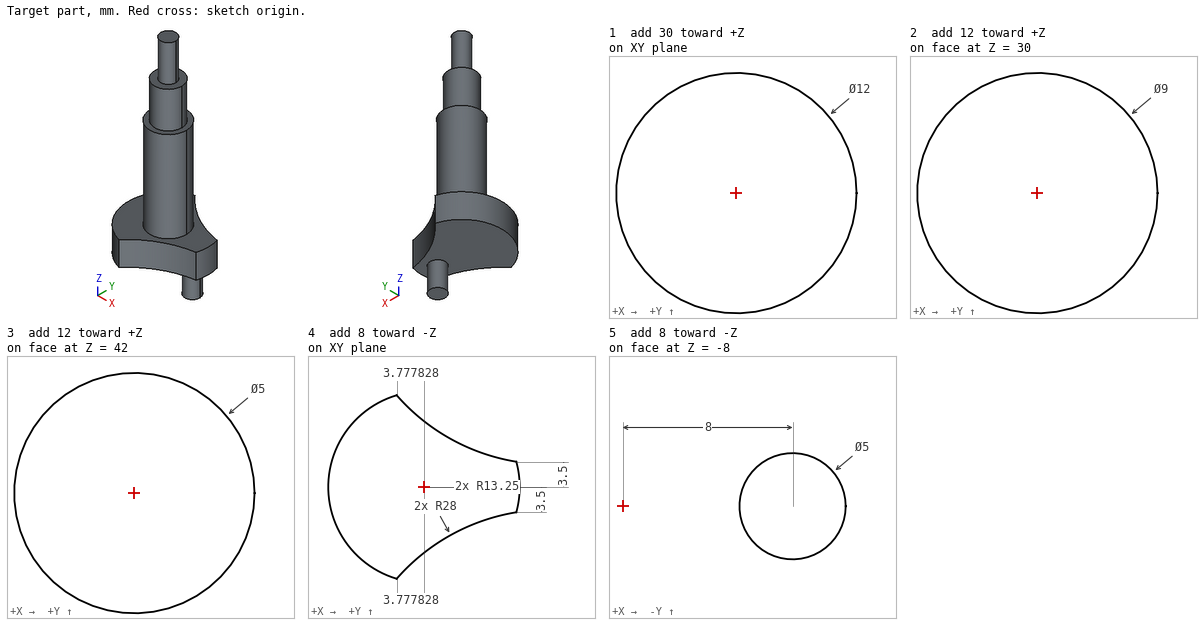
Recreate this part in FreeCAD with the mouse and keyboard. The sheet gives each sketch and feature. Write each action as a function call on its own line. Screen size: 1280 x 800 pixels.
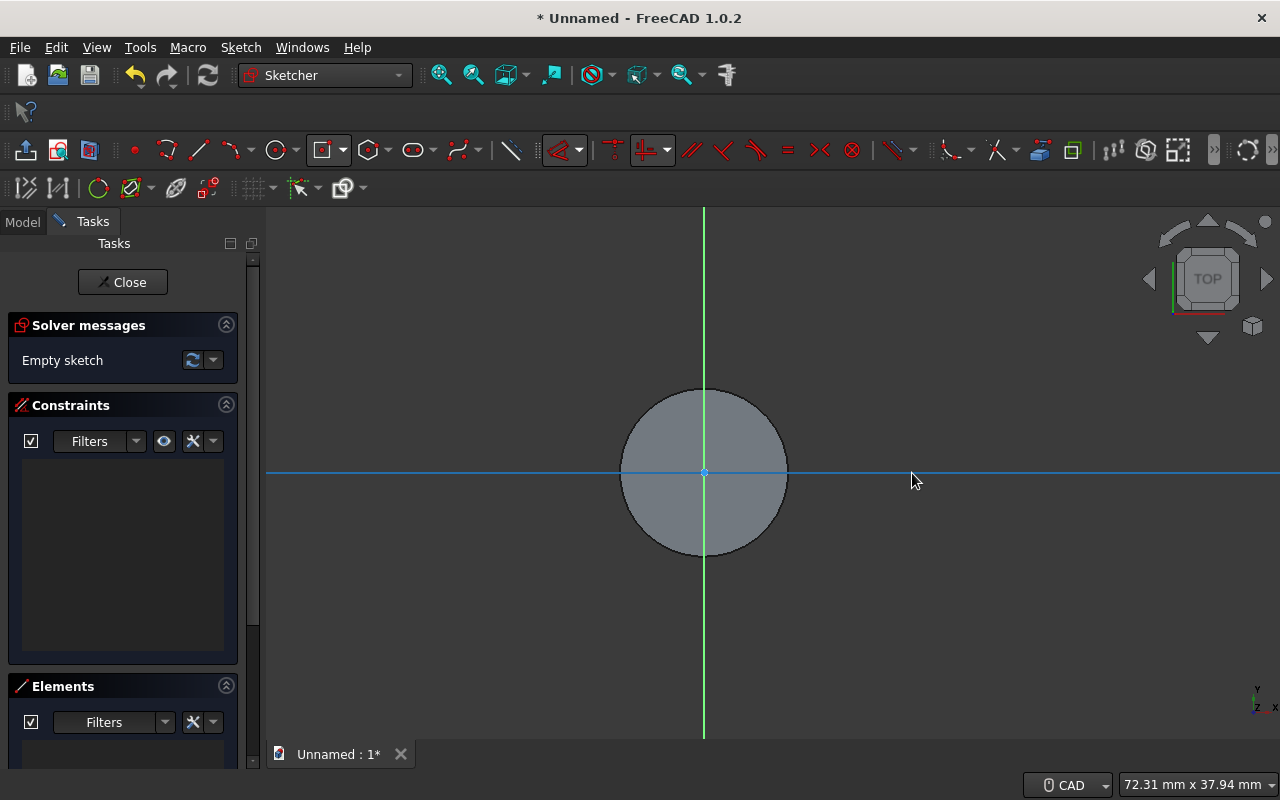
click(232, 150)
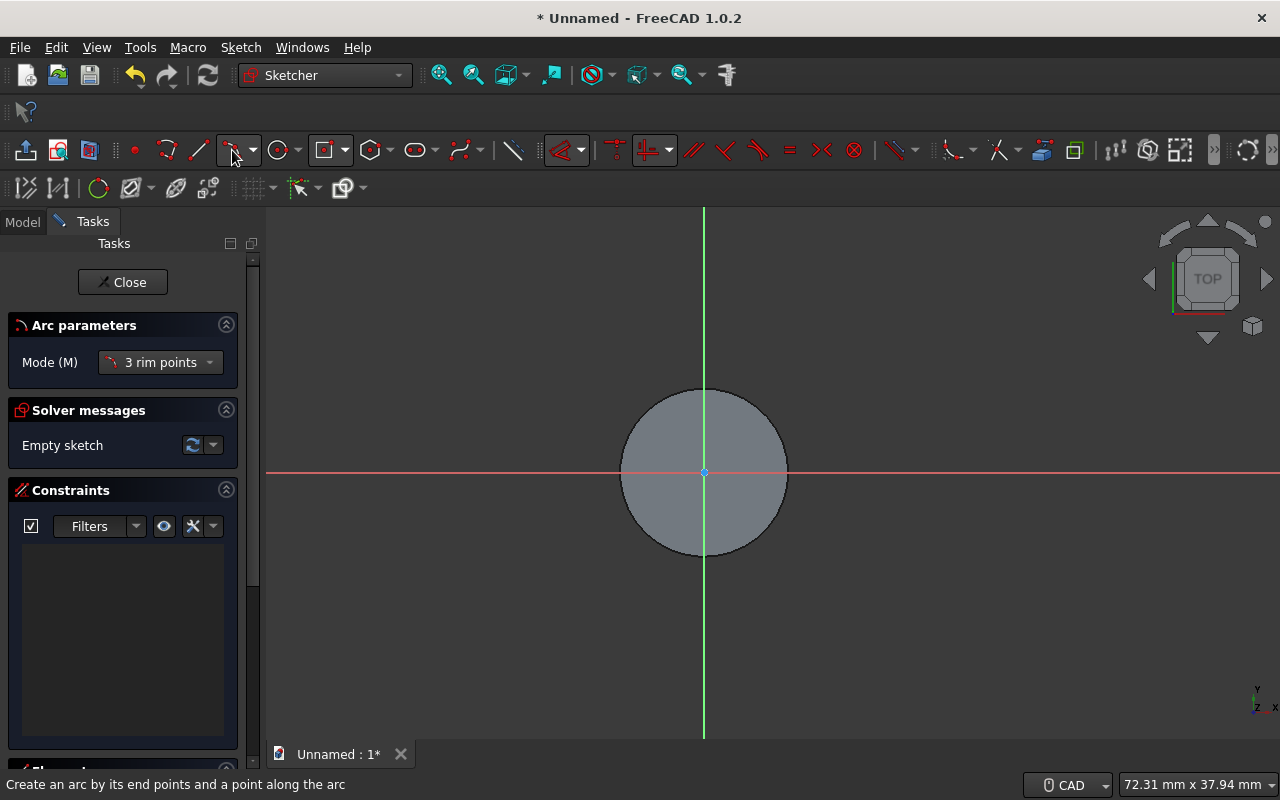
click(651, 651)
click(651, 295)
click(524, 426)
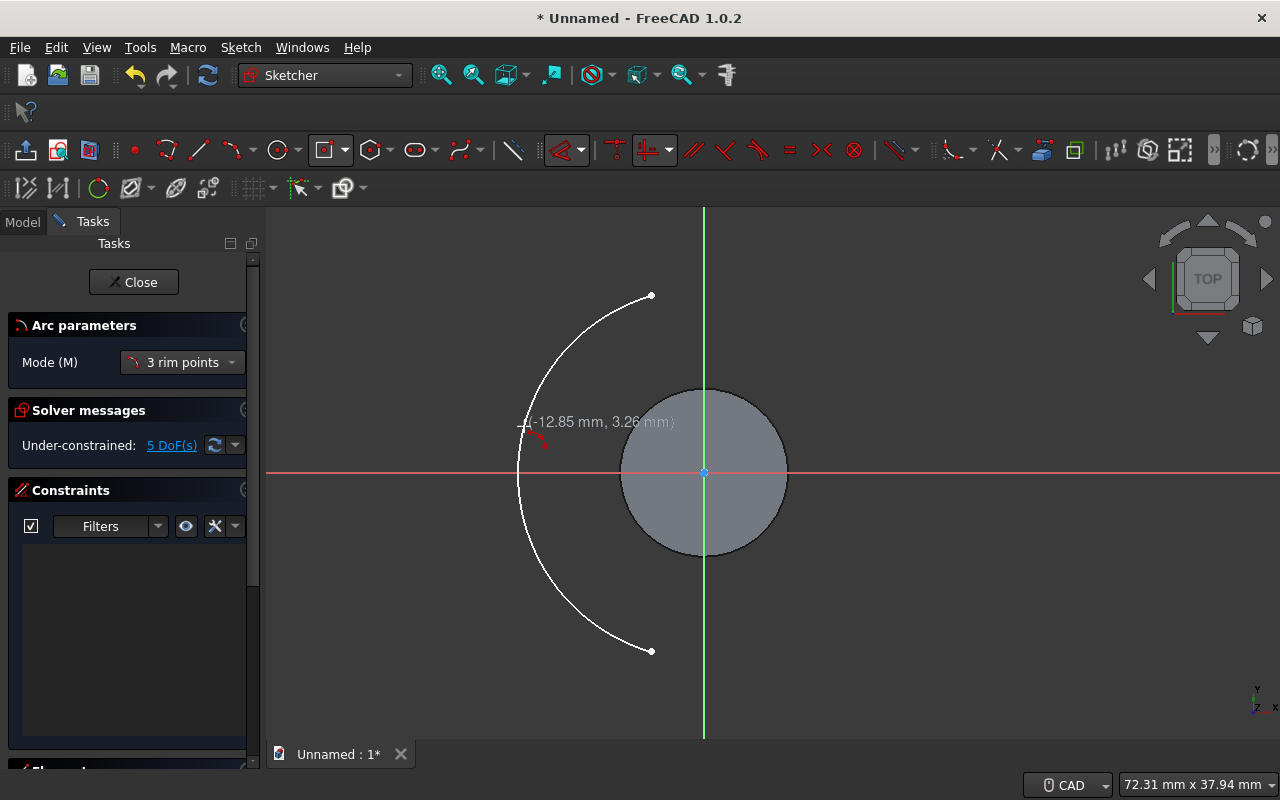
click(651, 296)
click(883, 424)
click(756, 379)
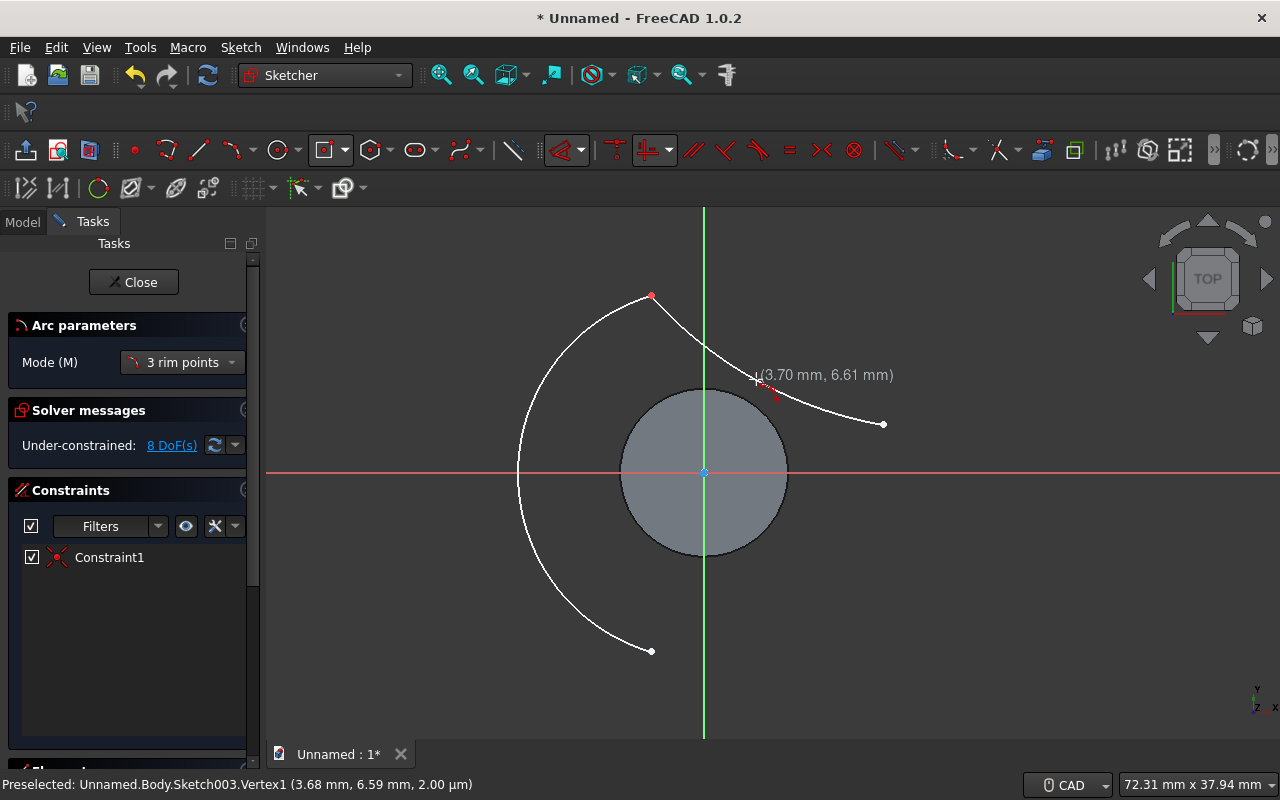
click(883, 425)
click(883, 522)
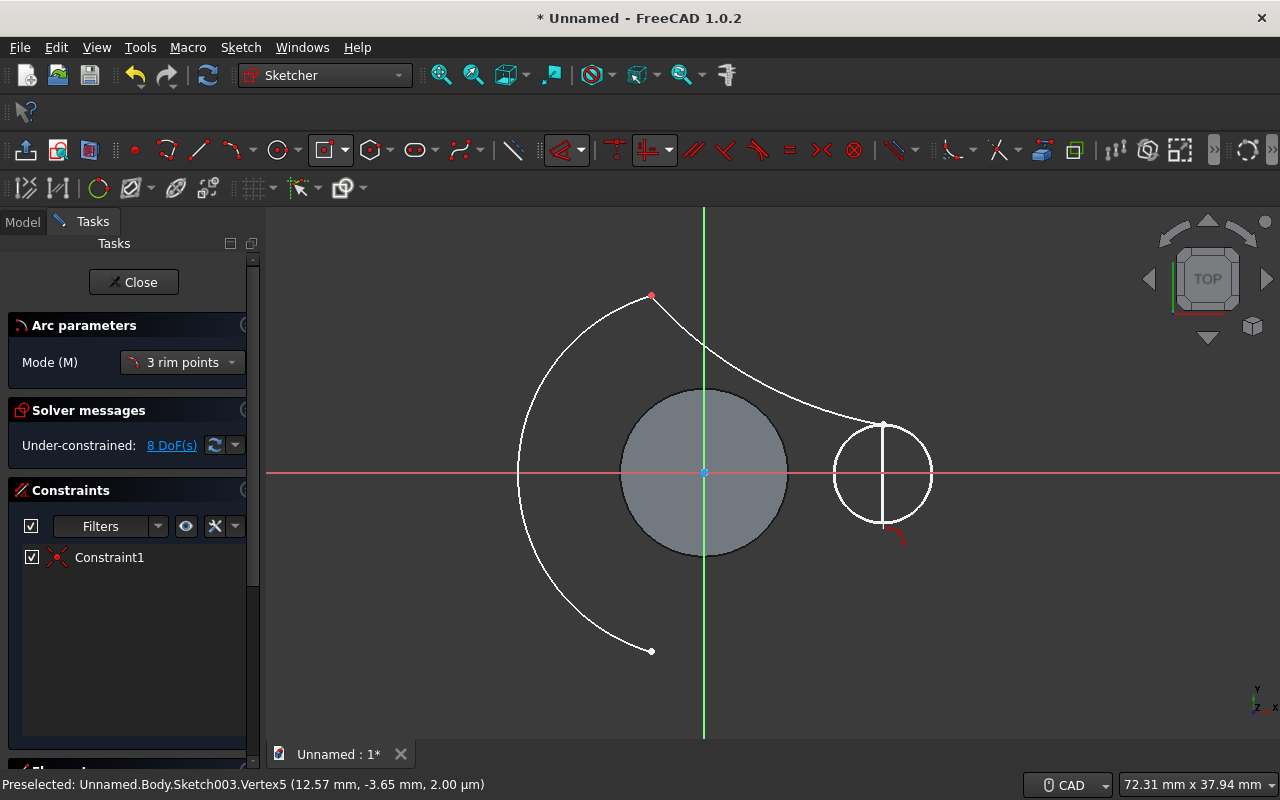
scroll(890, 483, up, 5)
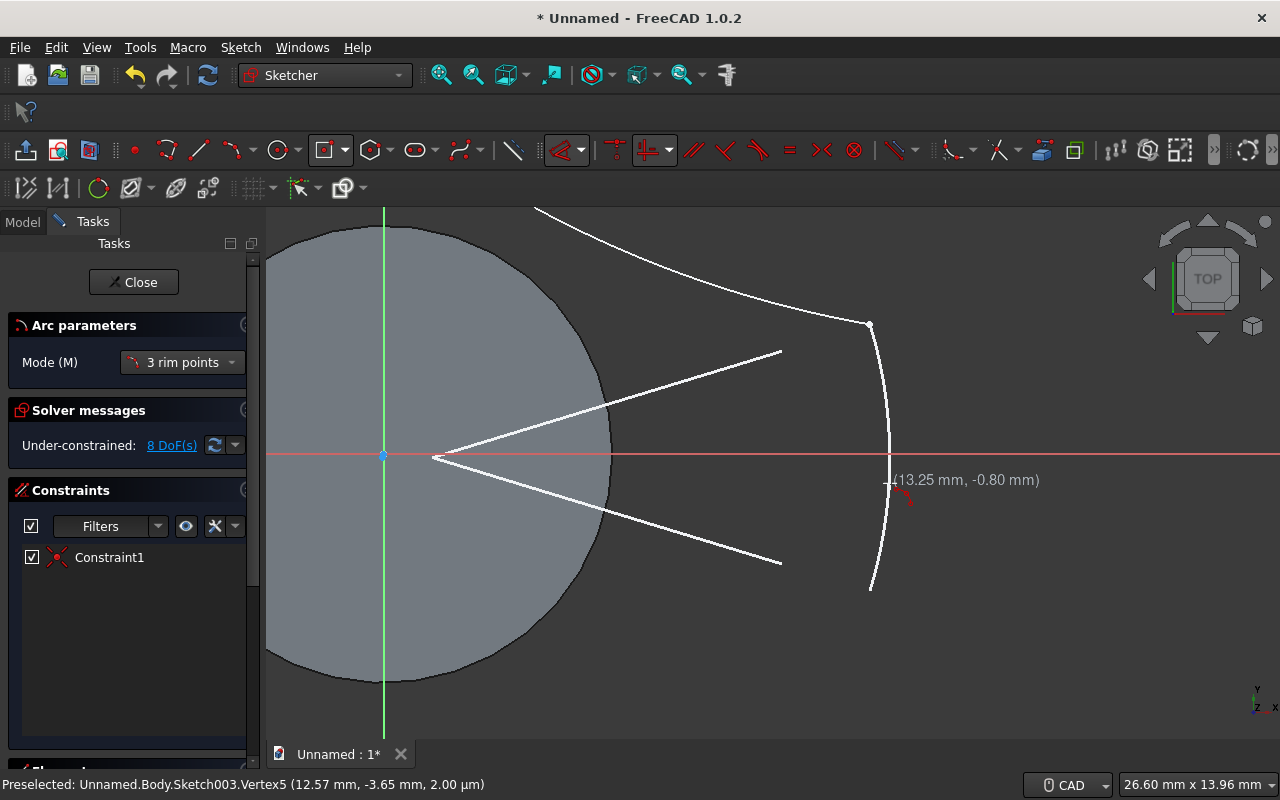
click(888, 481)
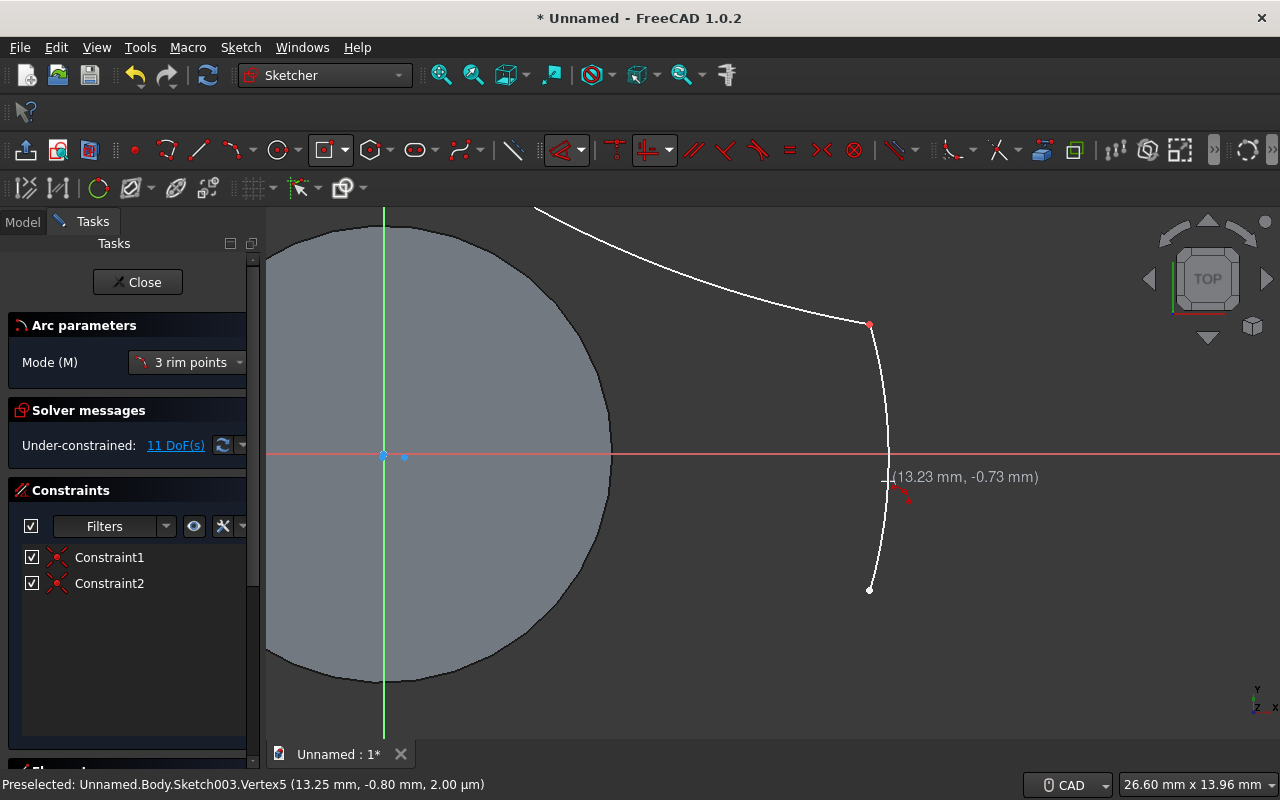
click(870, 591)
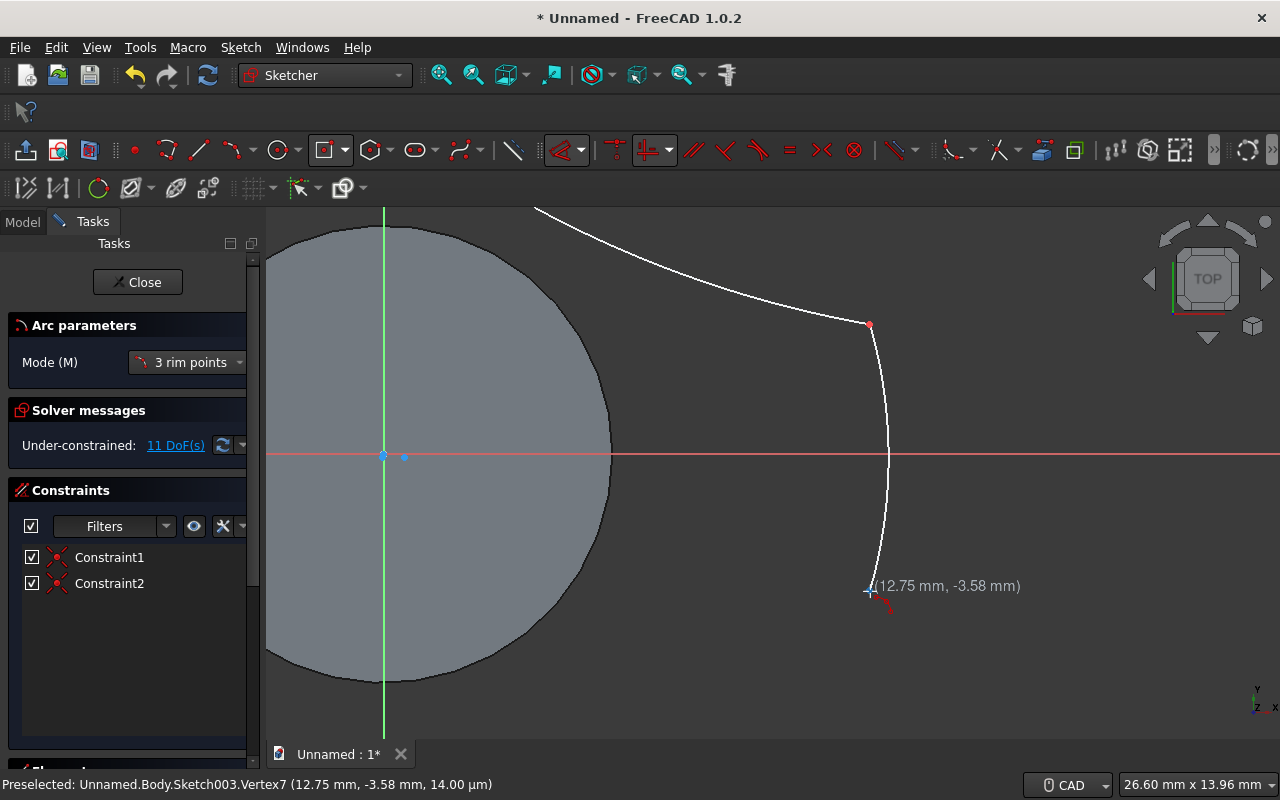
scroll(891, 484, down, 5)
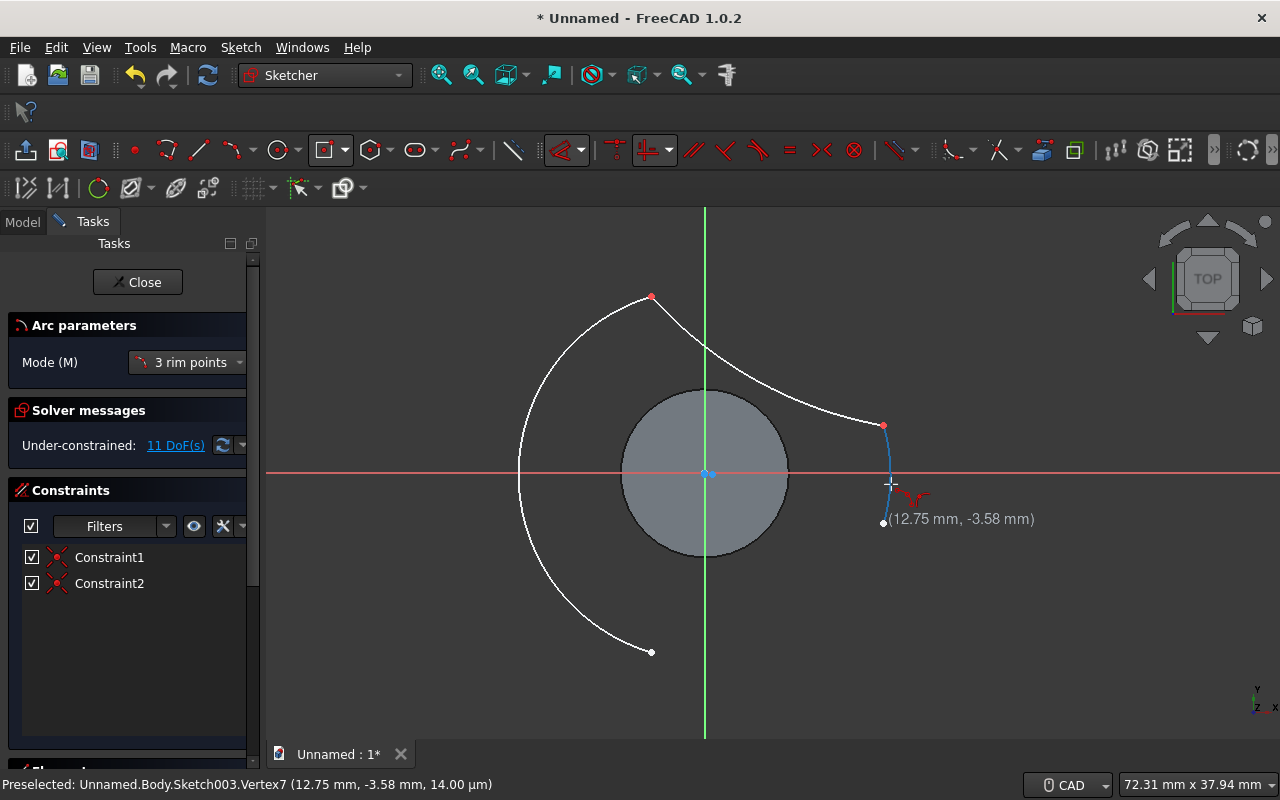
click(652, 653)
click(757, 567)
key(Escape)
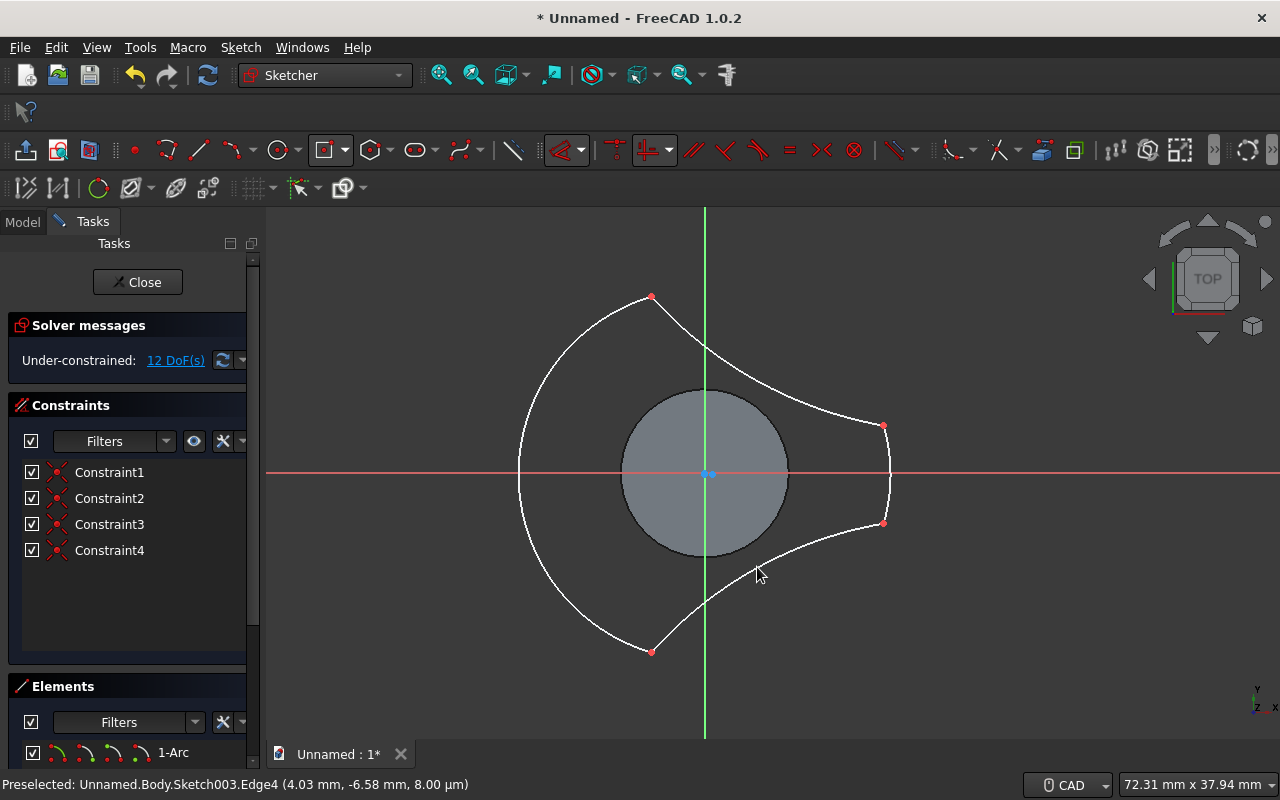
click(543, 383)